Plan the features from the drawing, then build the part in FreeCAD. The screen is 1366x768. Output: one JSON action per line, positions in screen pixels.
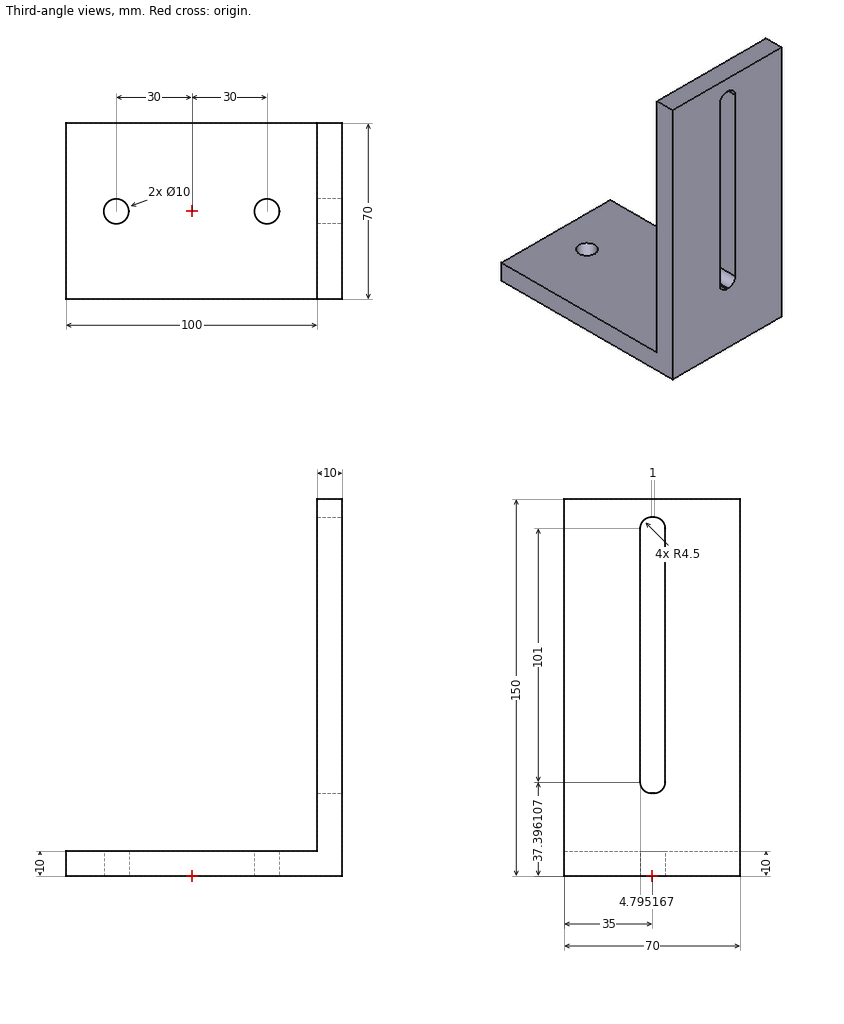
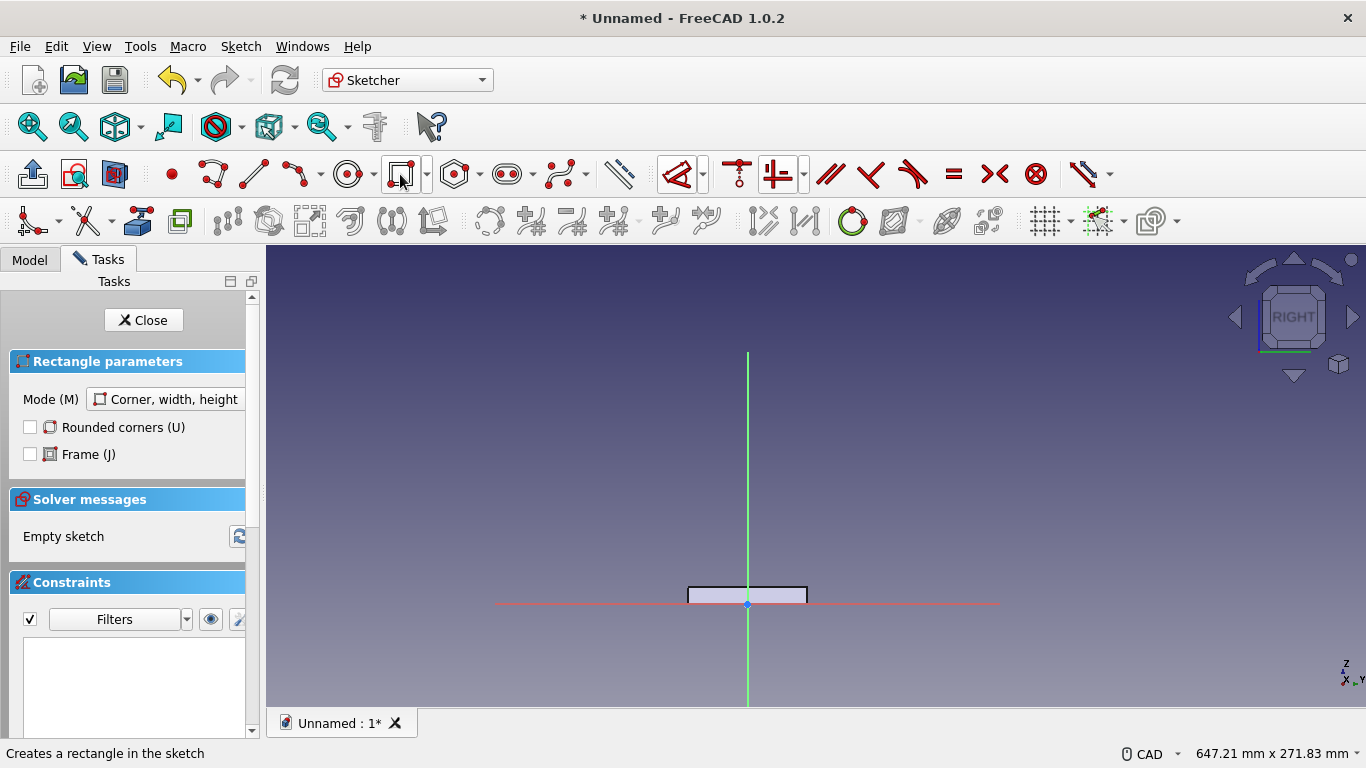
{"action": "left_click", "coordinate": [688, 349]}
{"action": "left_click", "coordinate": [807, 604]}
{"action": "key", "text": "Escape"}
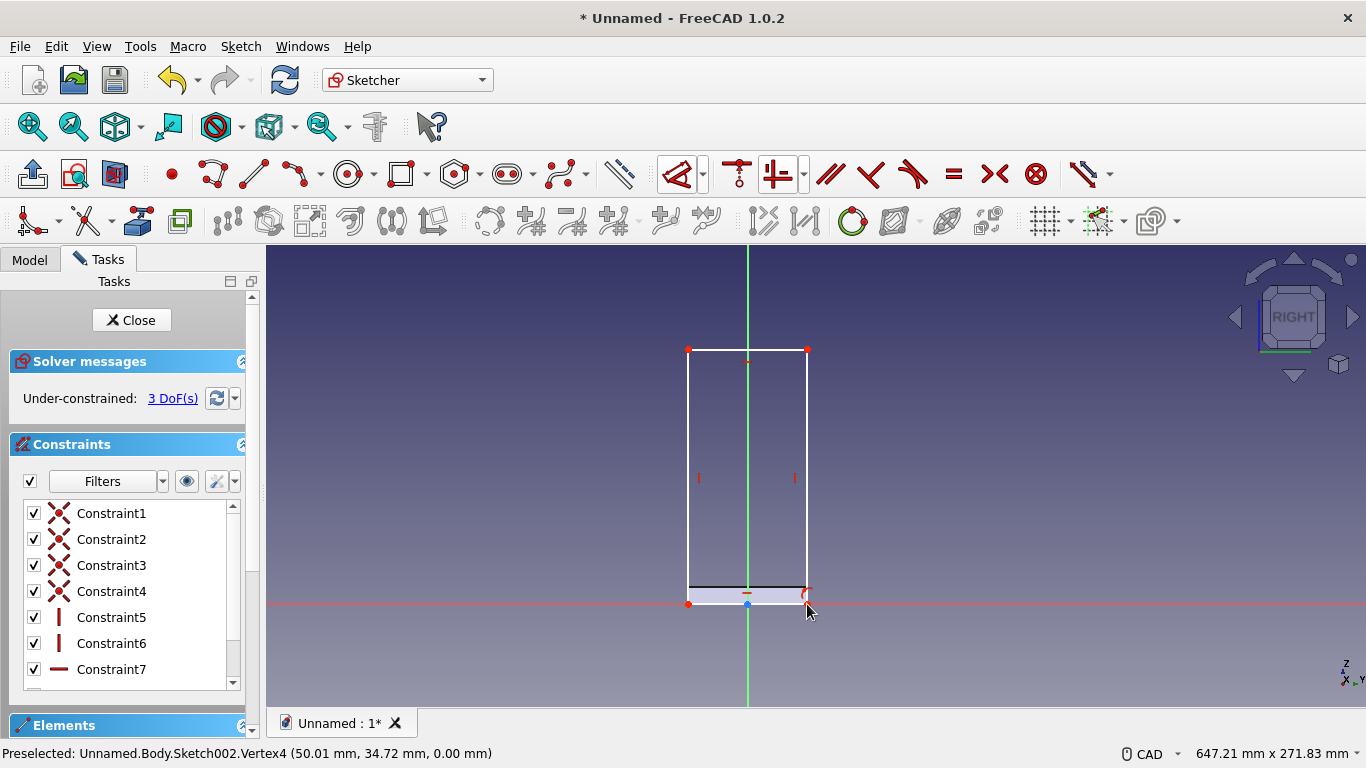
{"action": "left_click", "coordinate": [724, 604]}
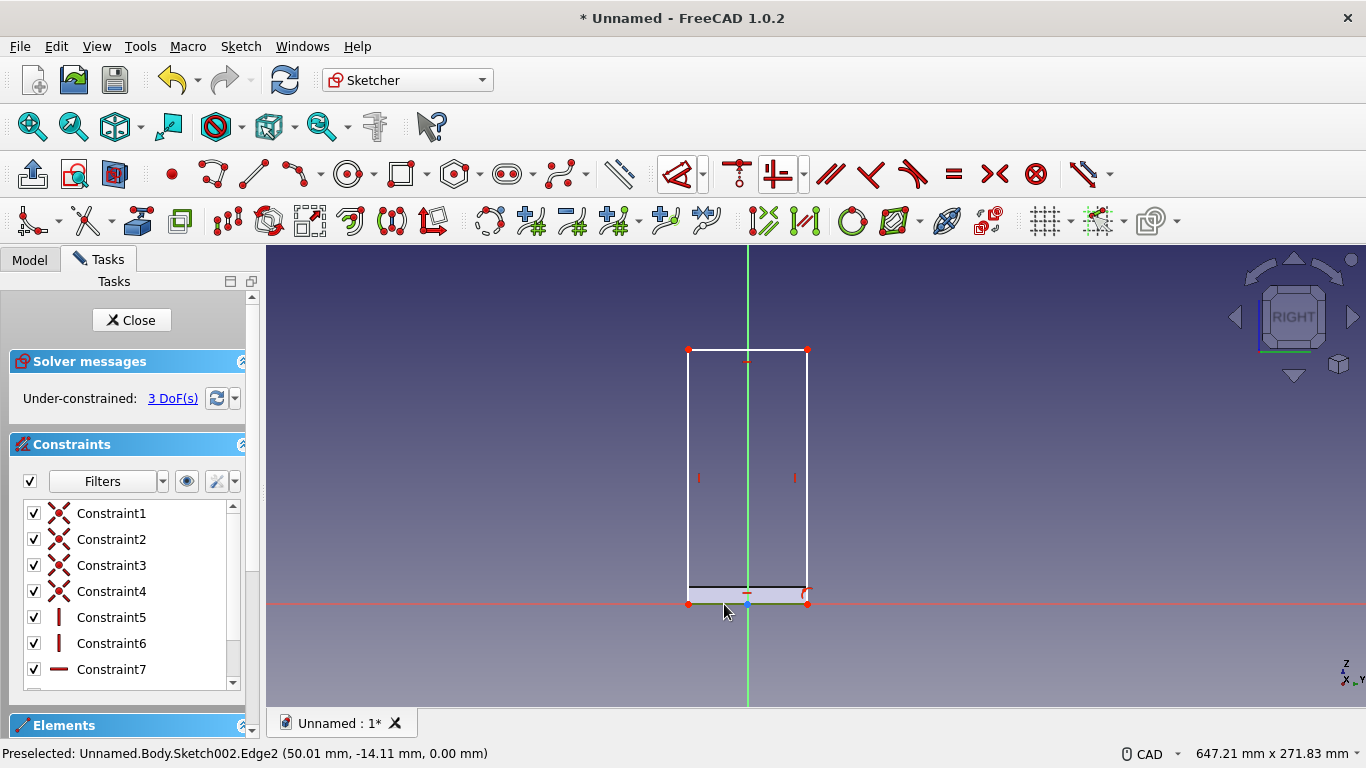
{"action": "key", "text": "l"}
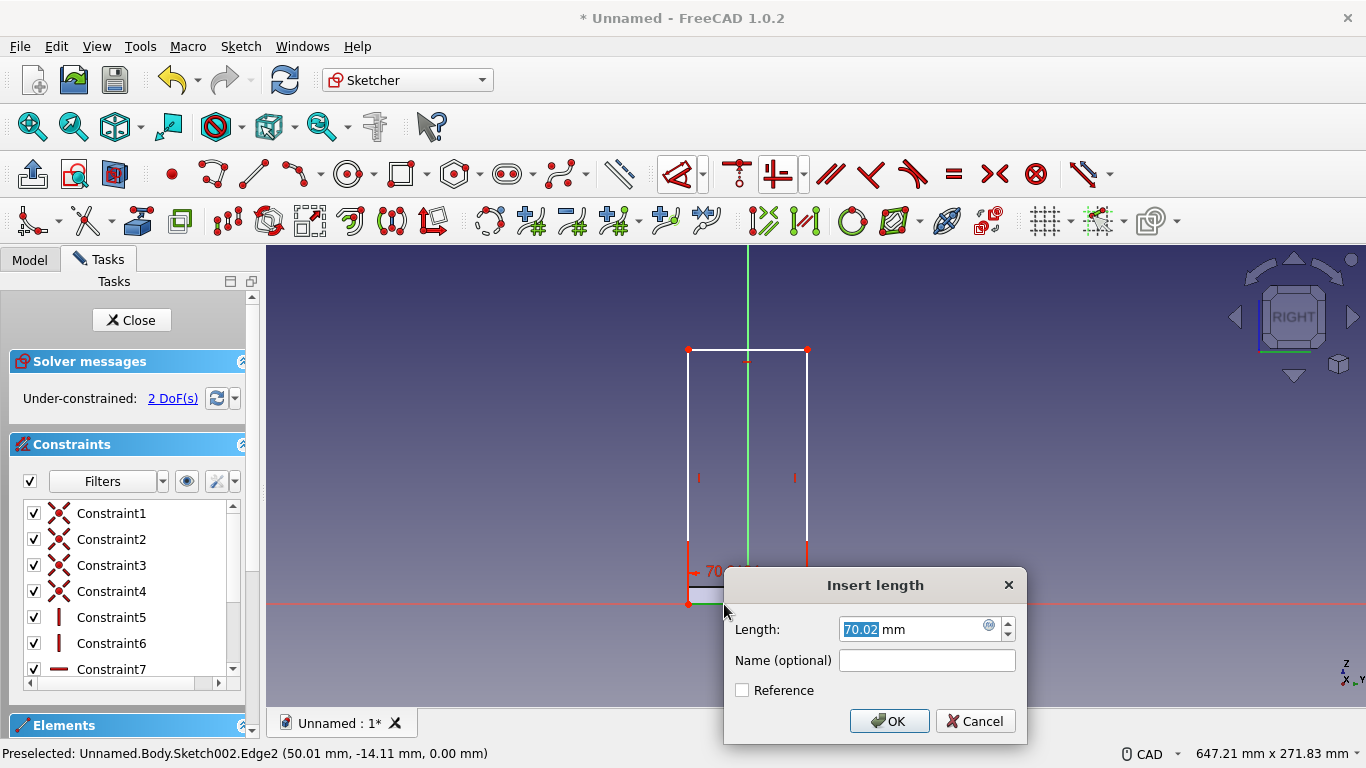
{"action": "type", "text": "70"}
{"action": "key", "text": "Return"}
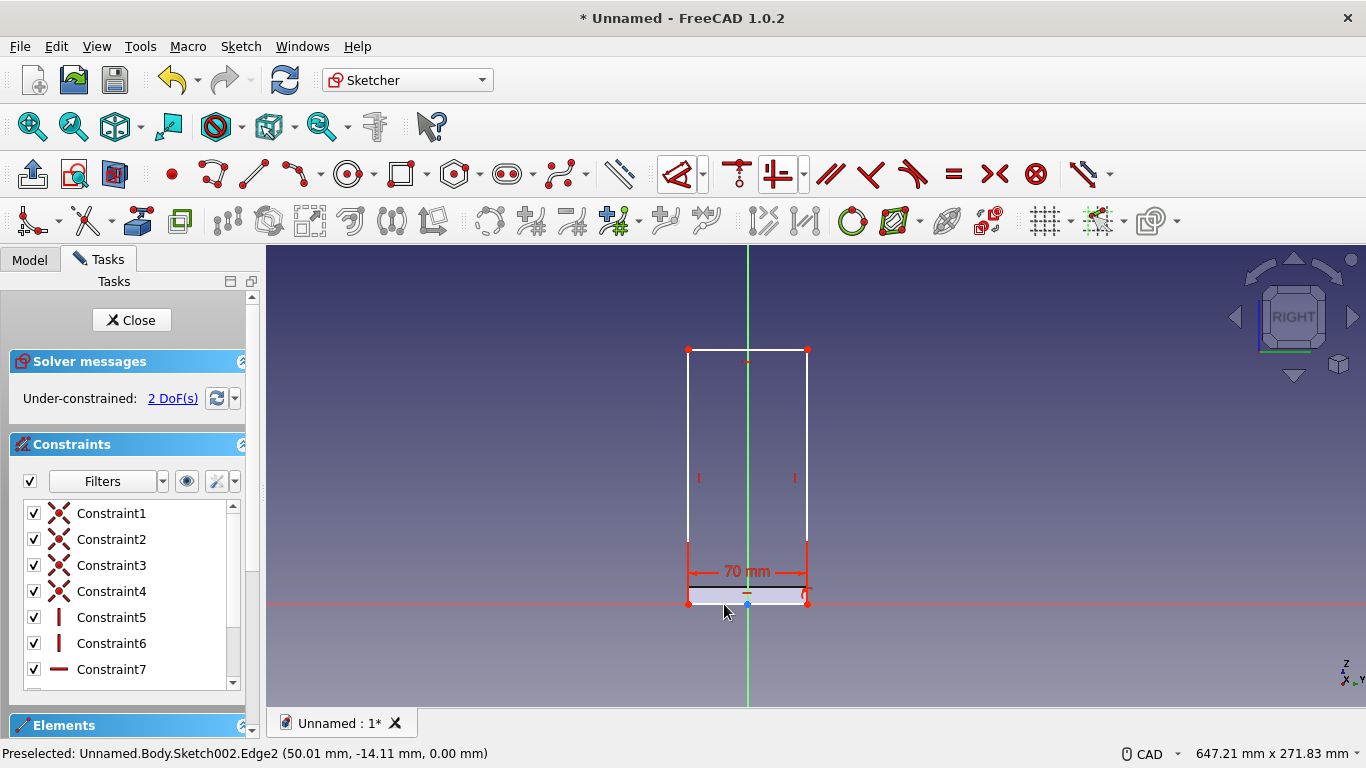
{"action": "left_click", "coordinate": [688, 426]}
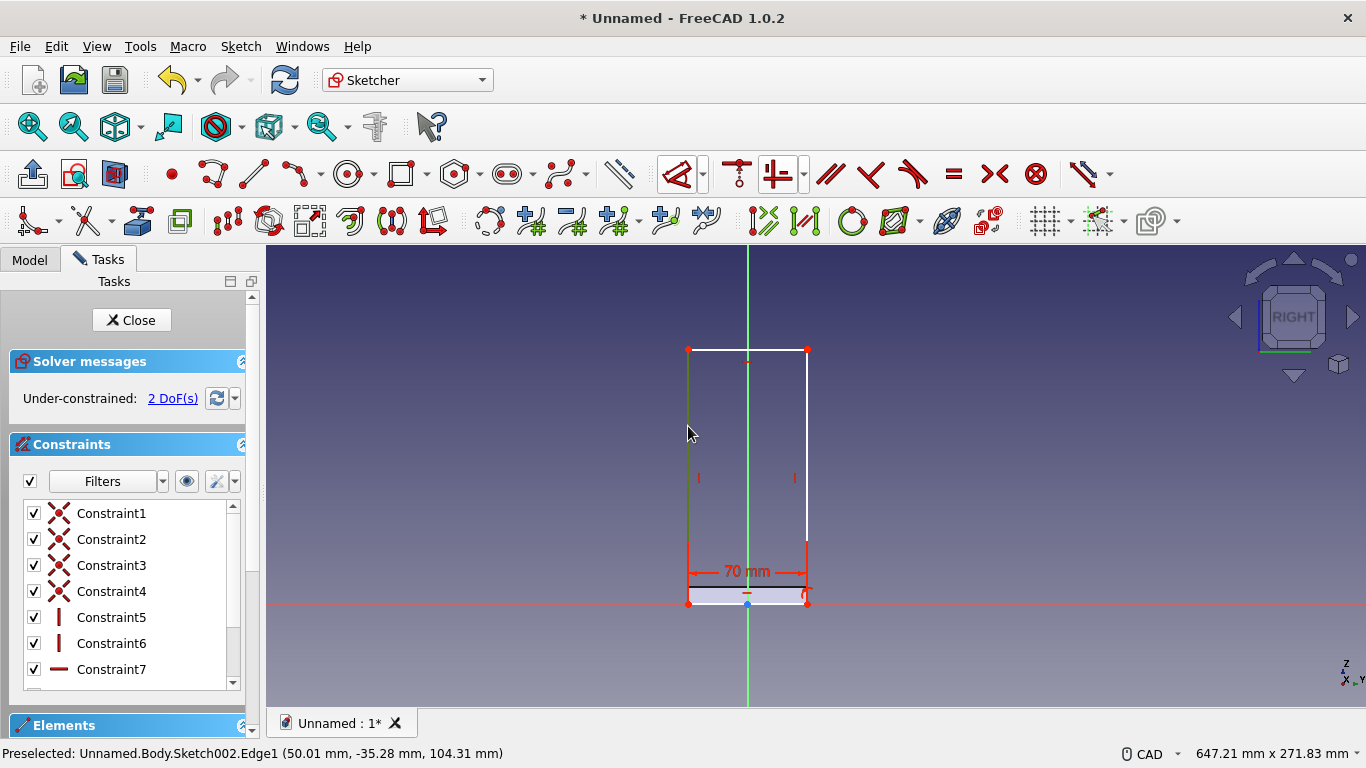
{"action": "key", "text": "i"}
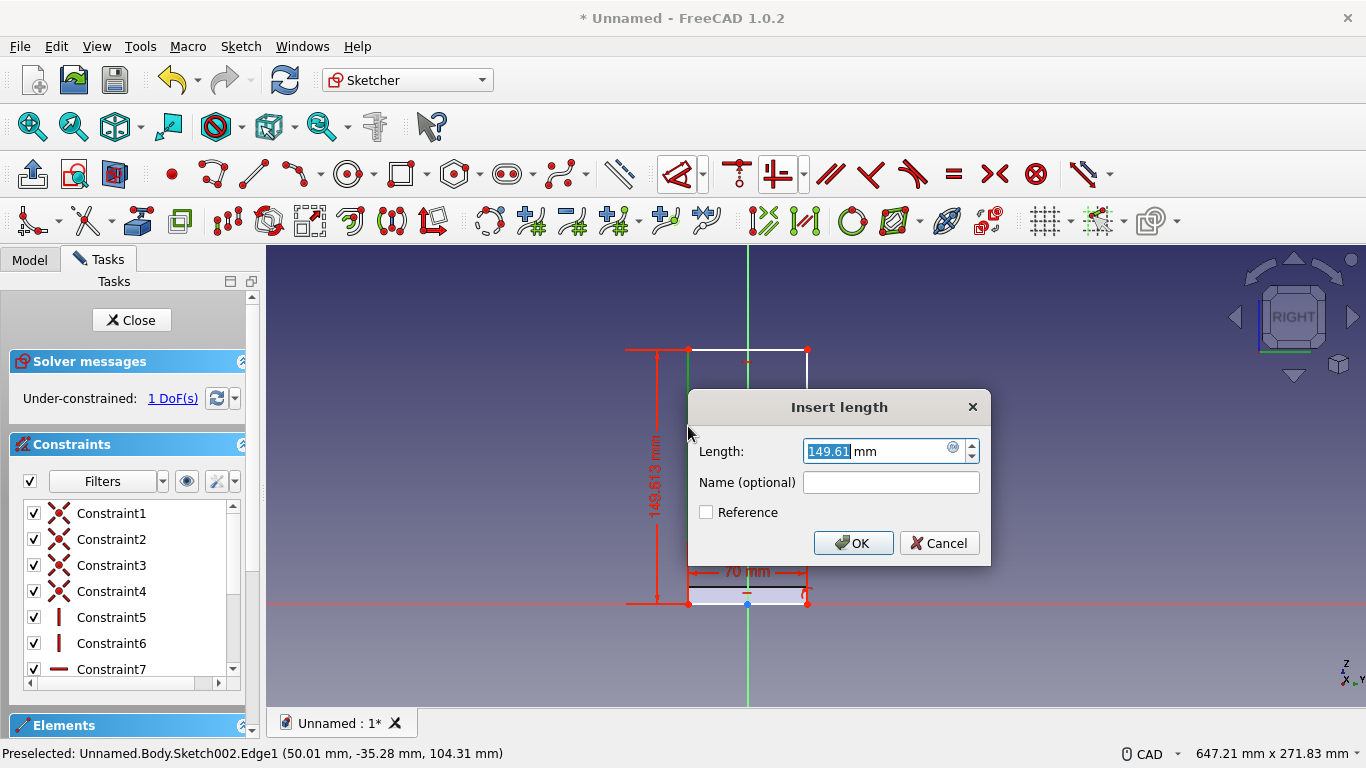
{"action": "type", "text": "150"}
{"action": "key", "text": "Return"}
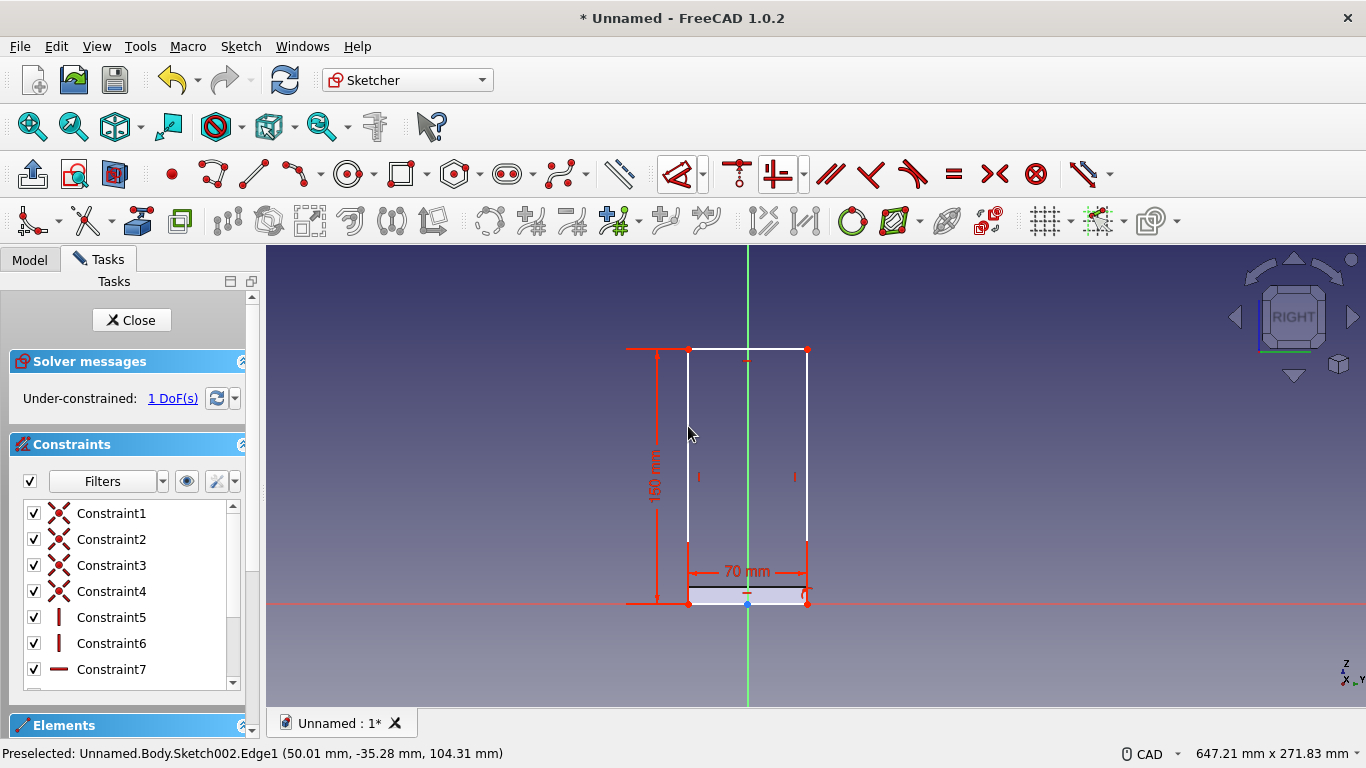
{"action": "left_click", "coordinate": [688, 349]}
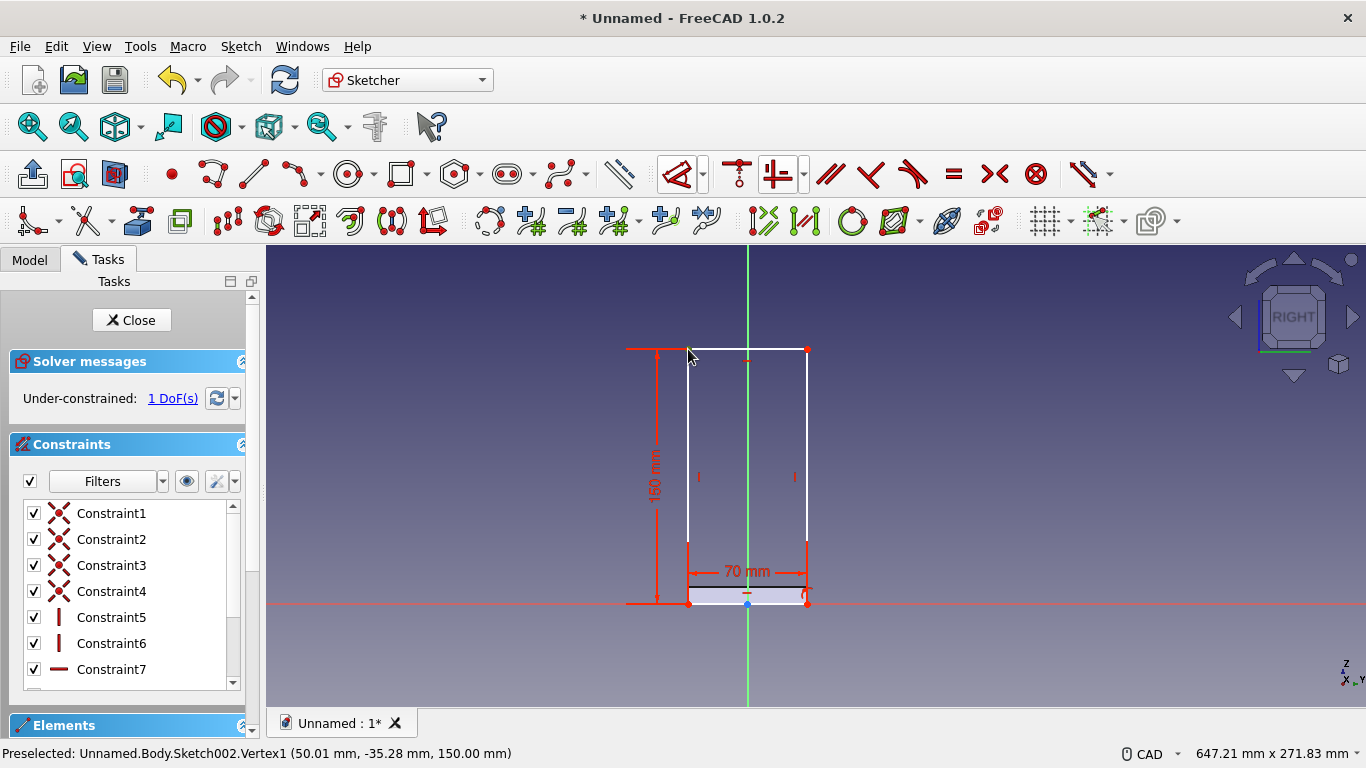
{"action": "key", "text": "l"}